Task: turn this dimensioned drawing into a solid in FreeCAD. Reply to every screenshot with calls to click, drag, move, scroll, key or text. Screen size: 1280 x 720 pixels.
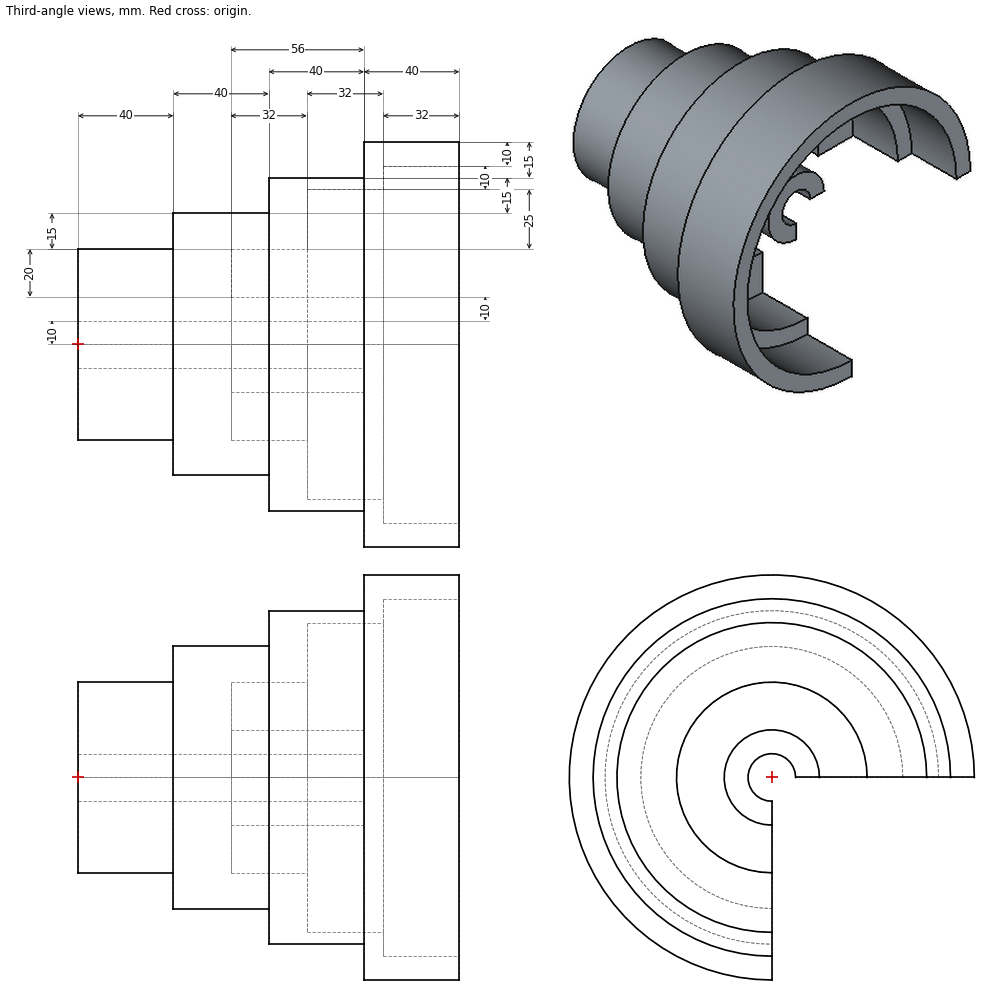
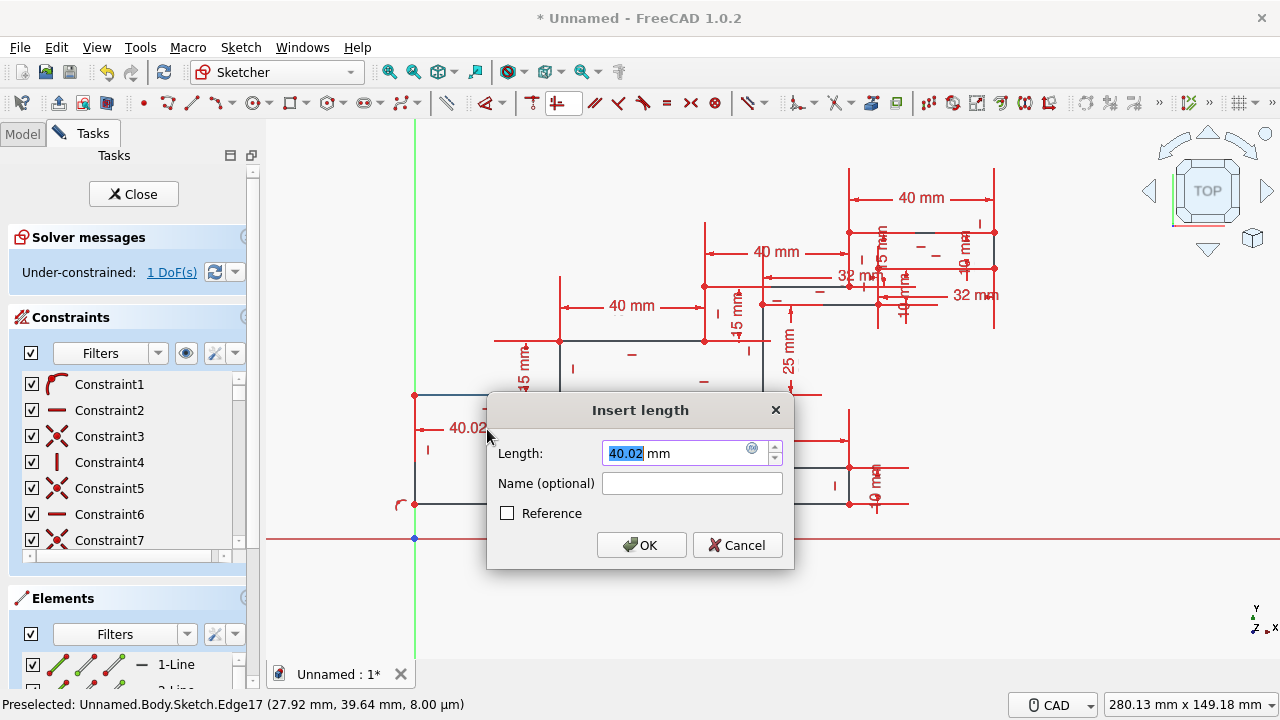
text(40)
key(Return)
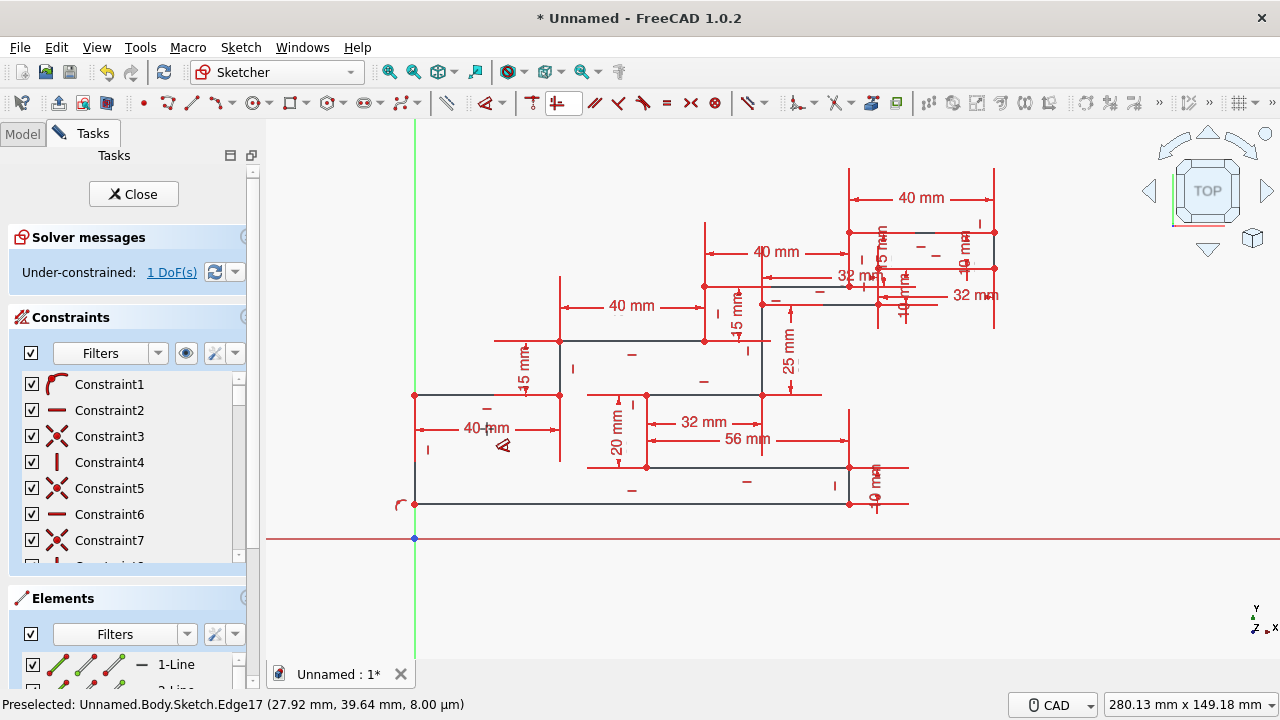
click(415, 504)
click(381, 521)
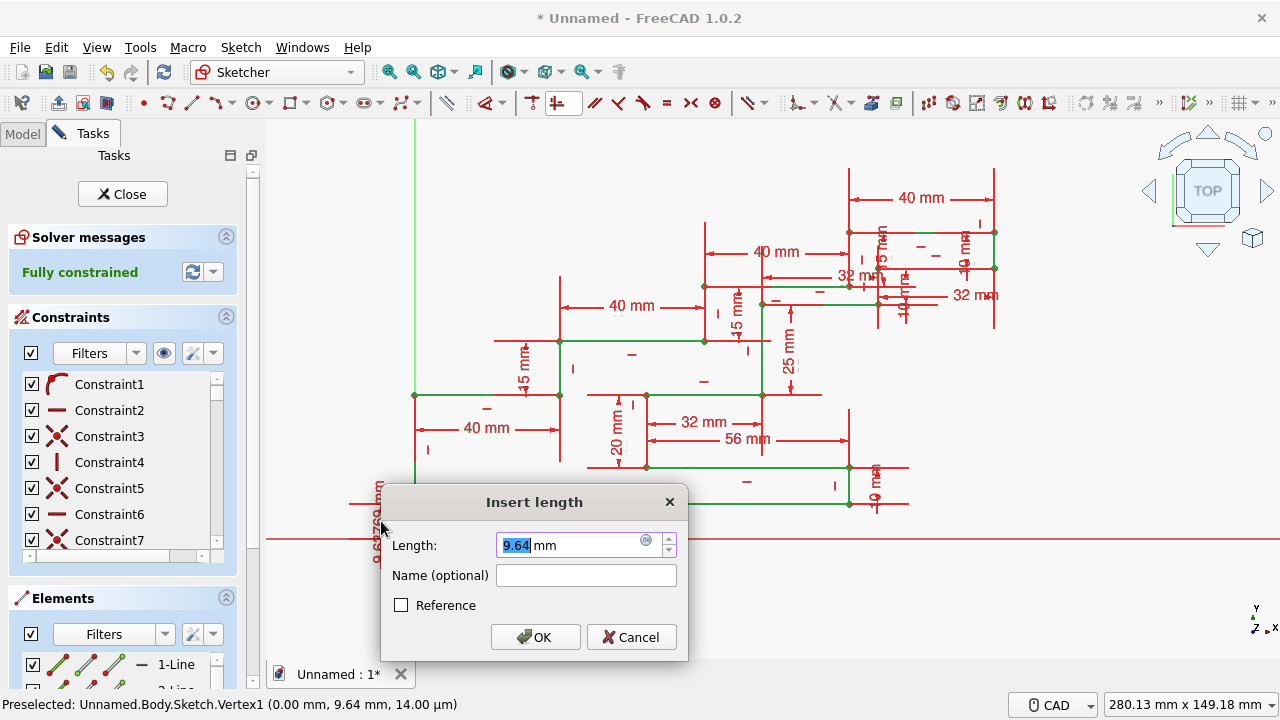
text(10)
key(Return)
key(Escape)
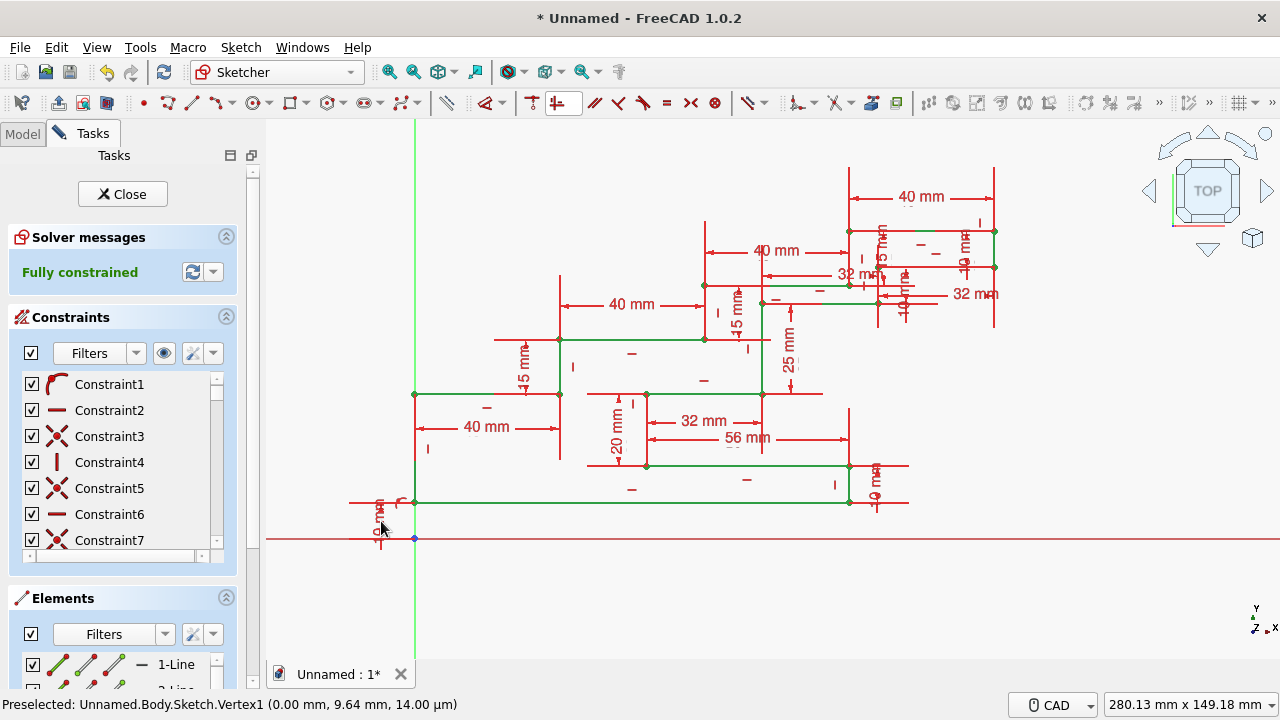
click(123, 194)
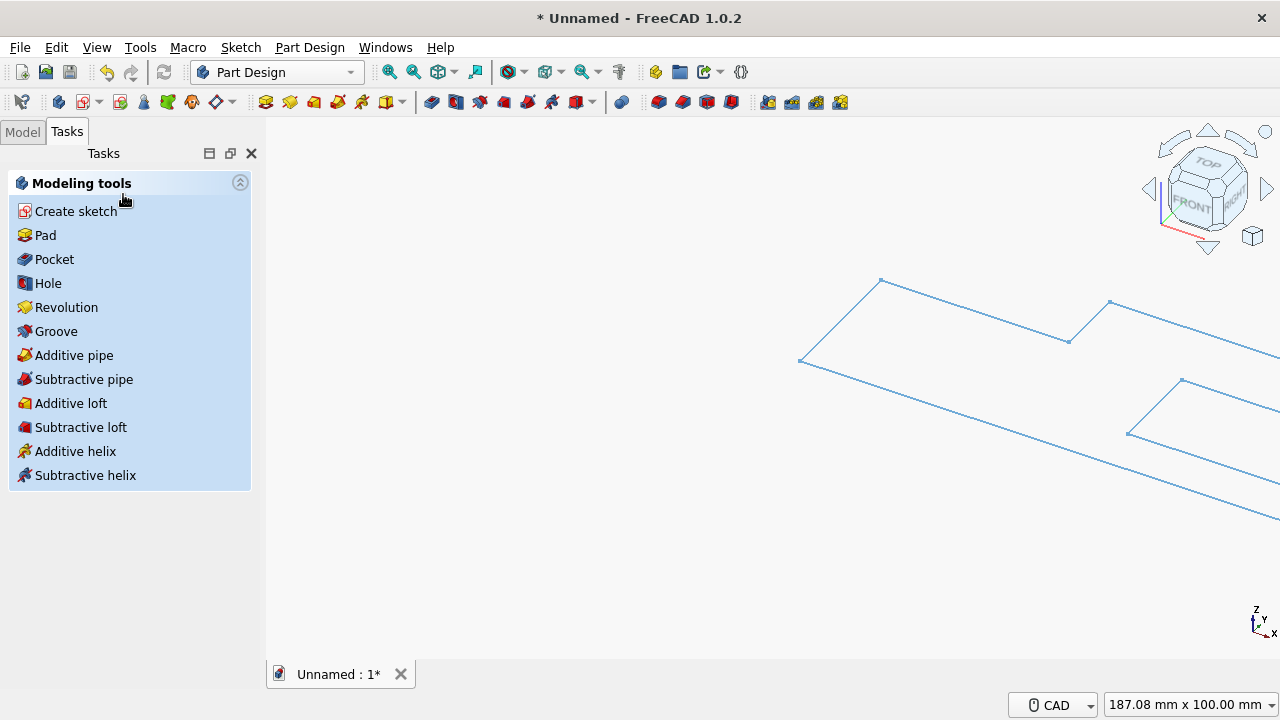
click(290, 102)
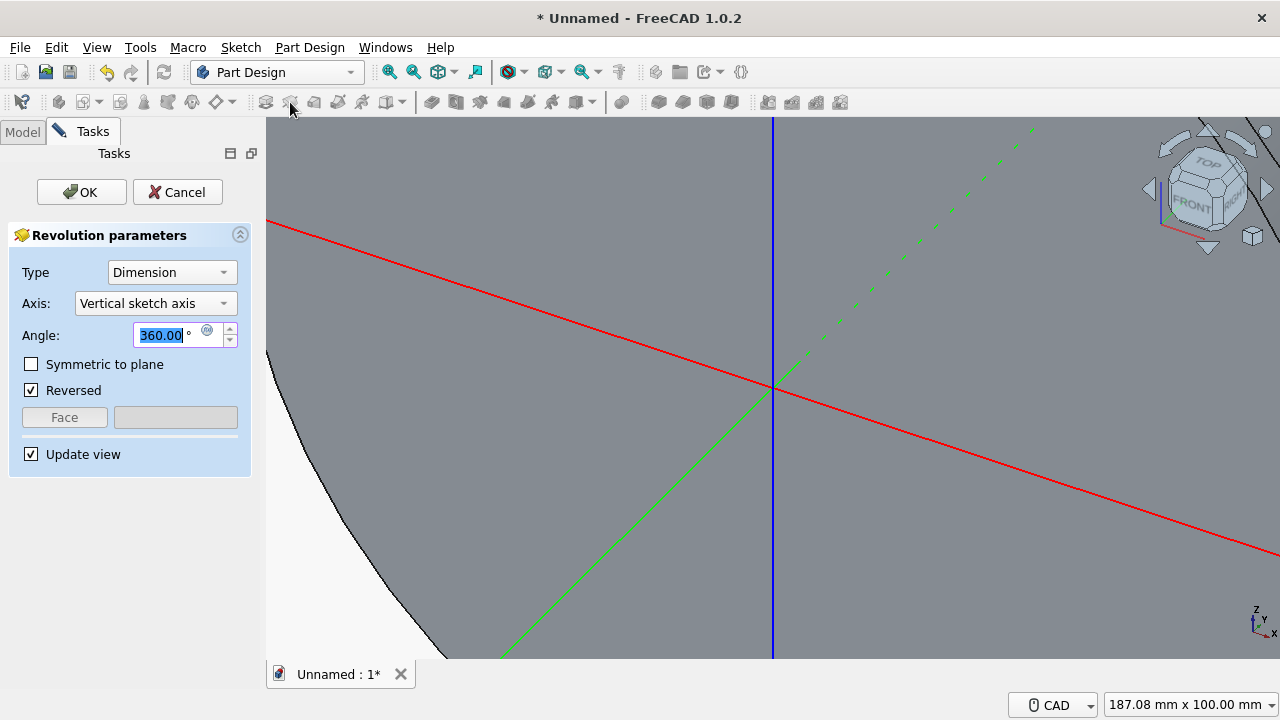
click(156, 304)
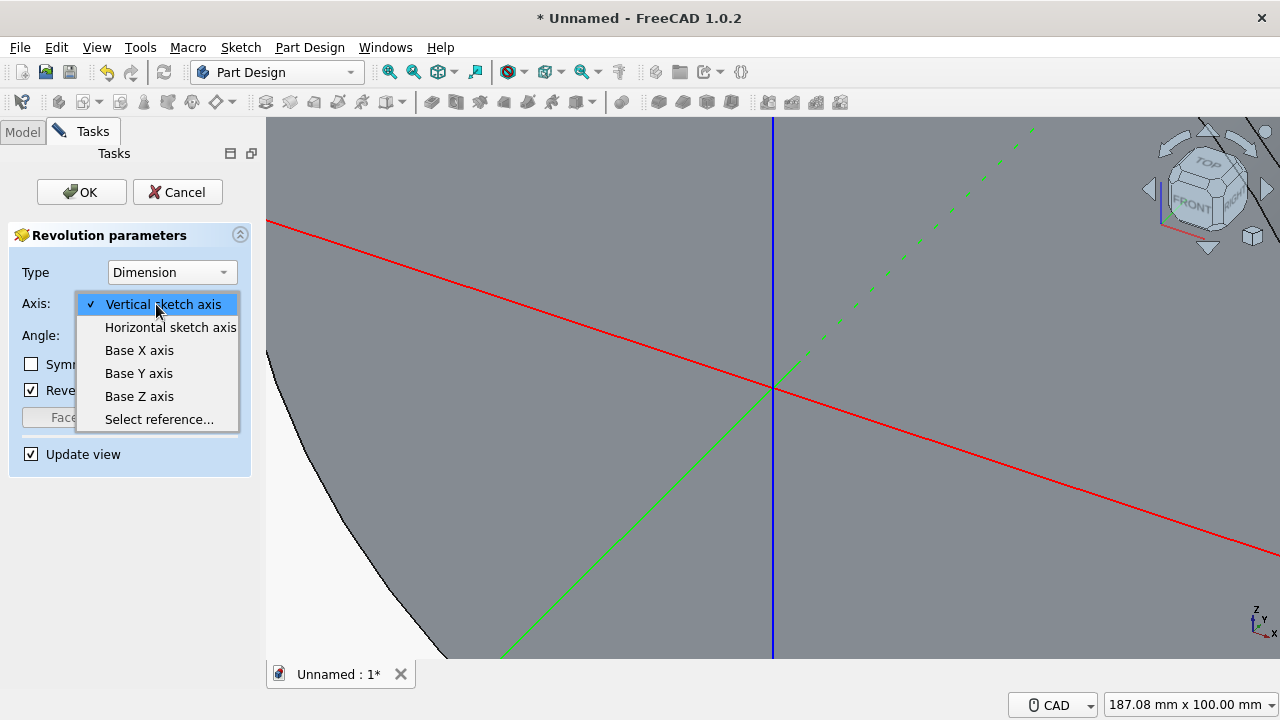
click(156, 328)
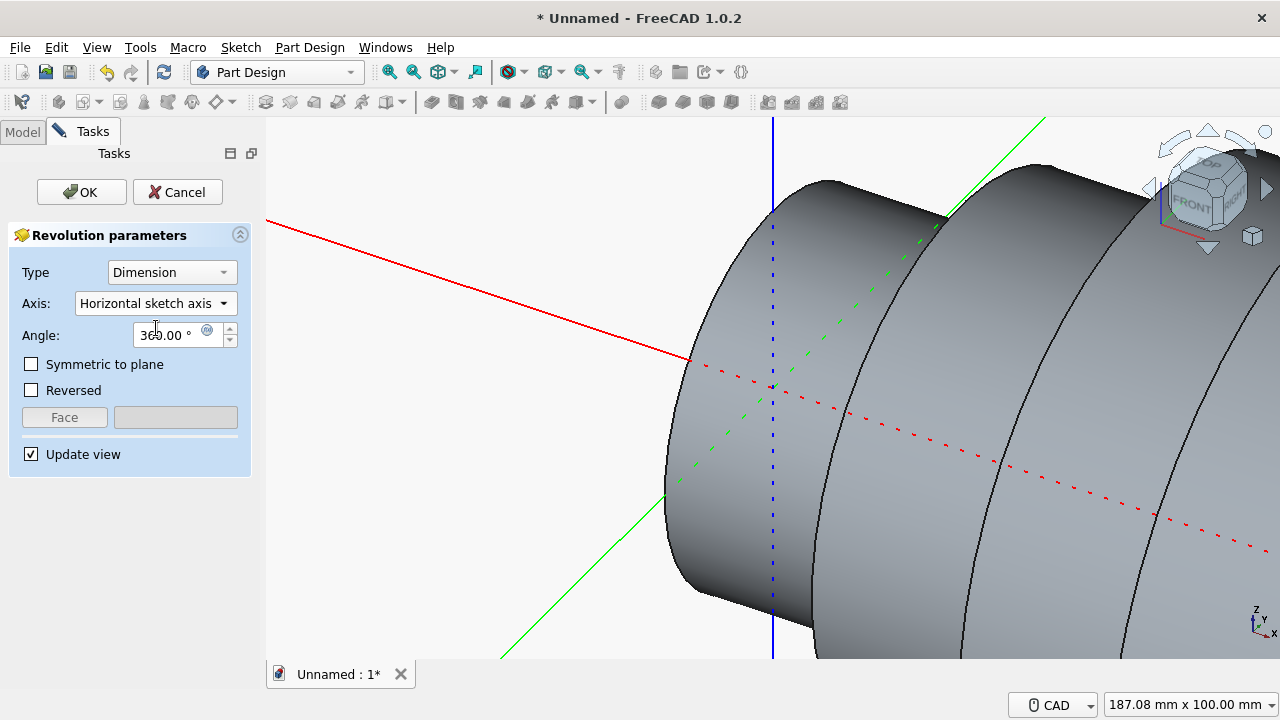
triple_click(178, 335)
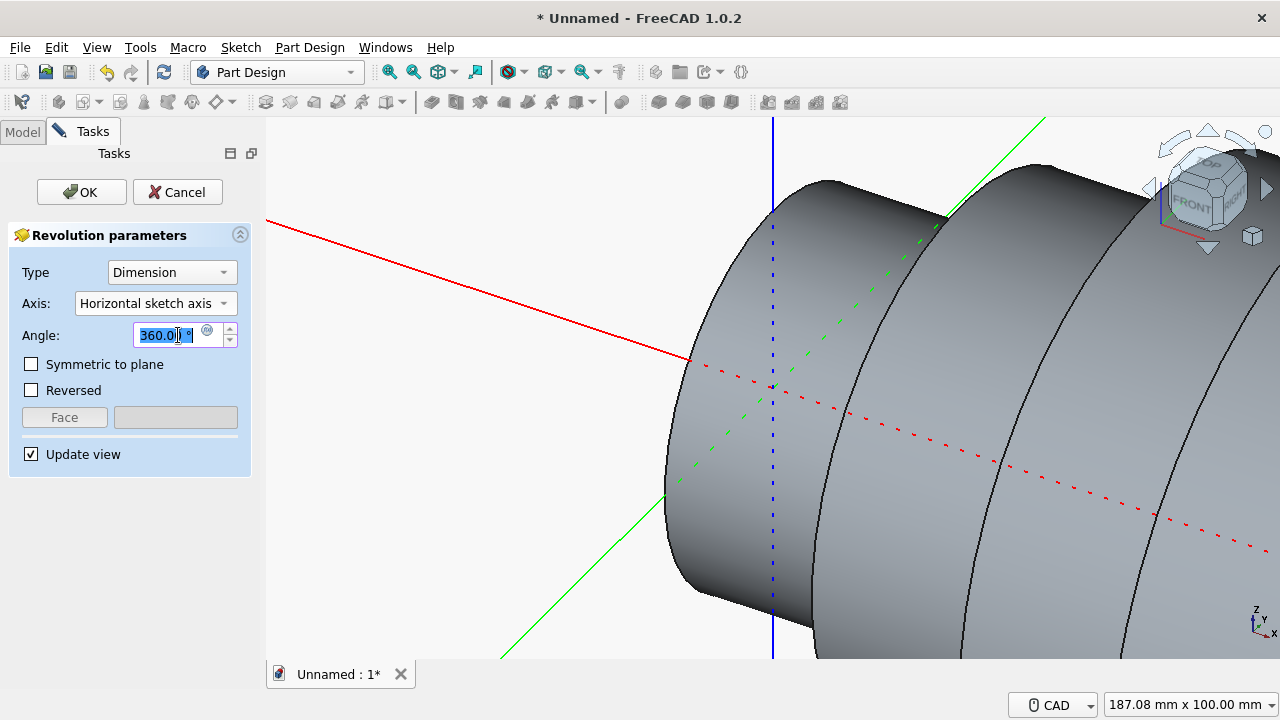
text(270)
key(Tab)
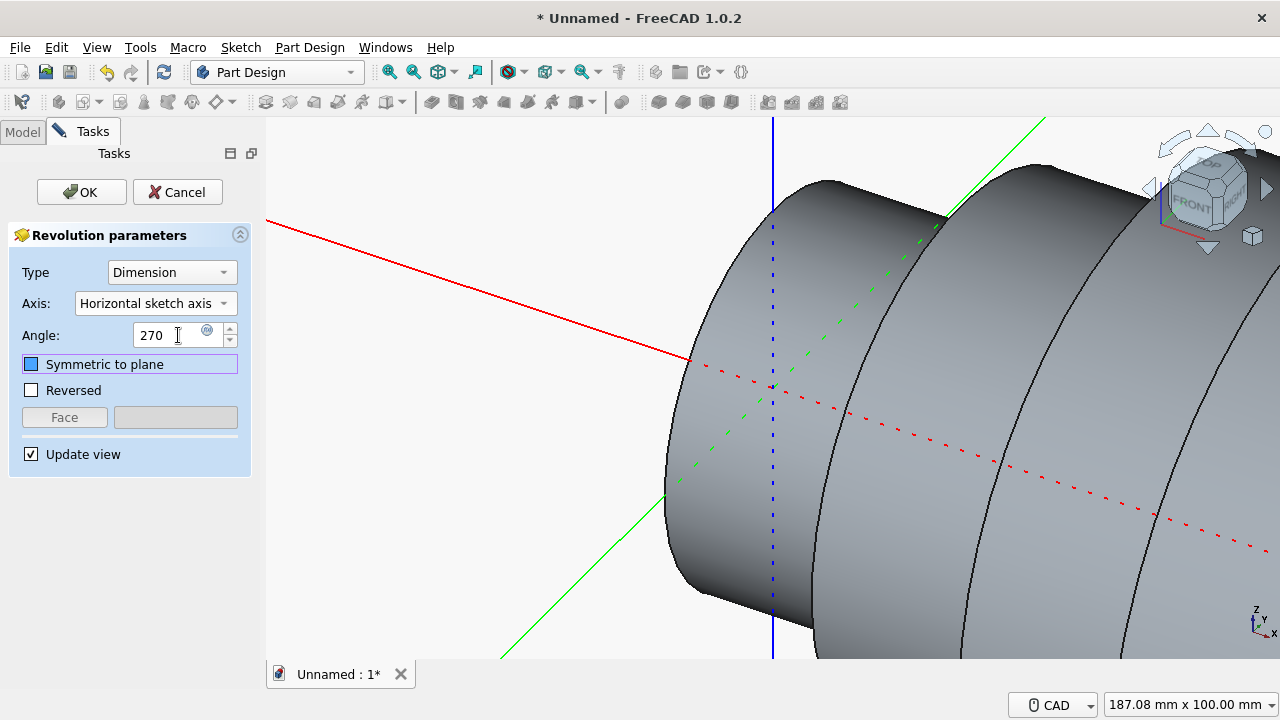
click(82, 192)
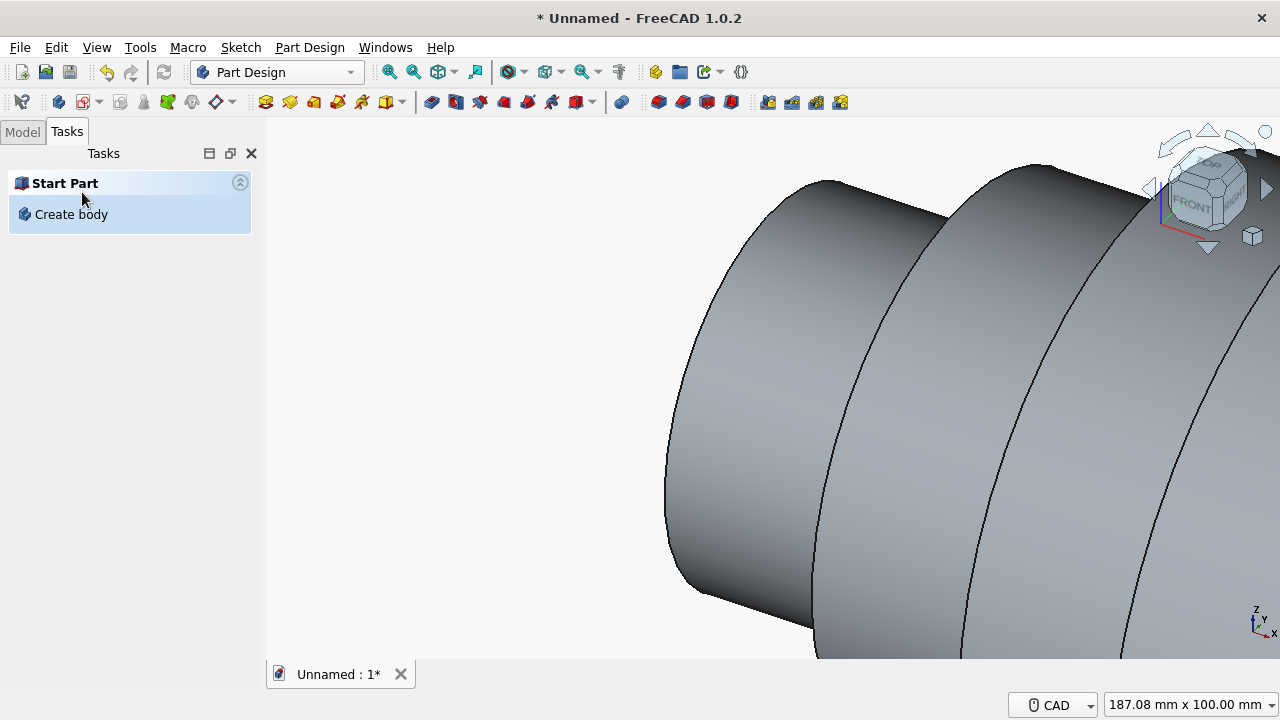
key(0)